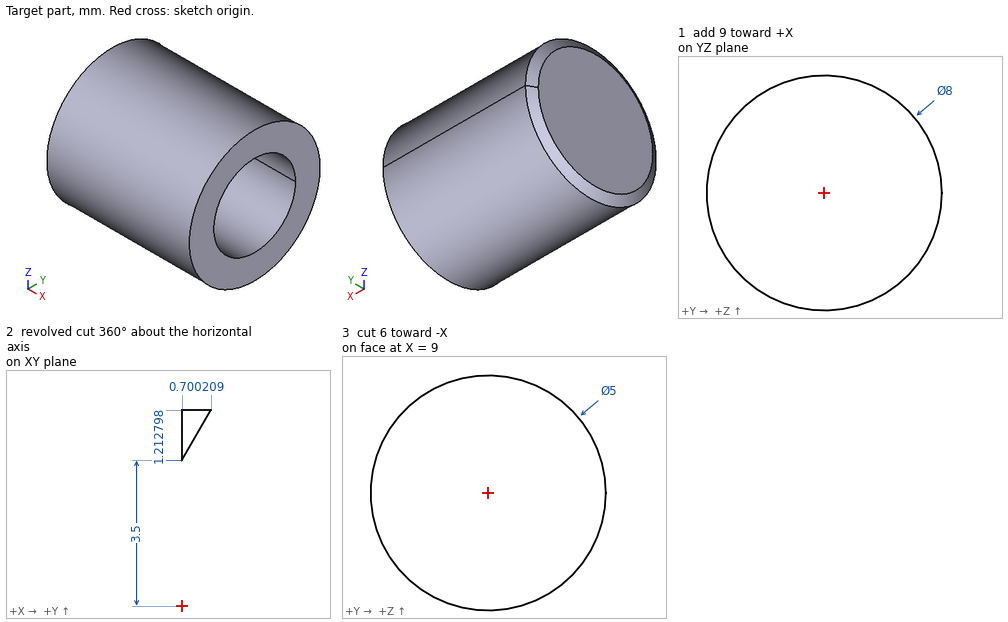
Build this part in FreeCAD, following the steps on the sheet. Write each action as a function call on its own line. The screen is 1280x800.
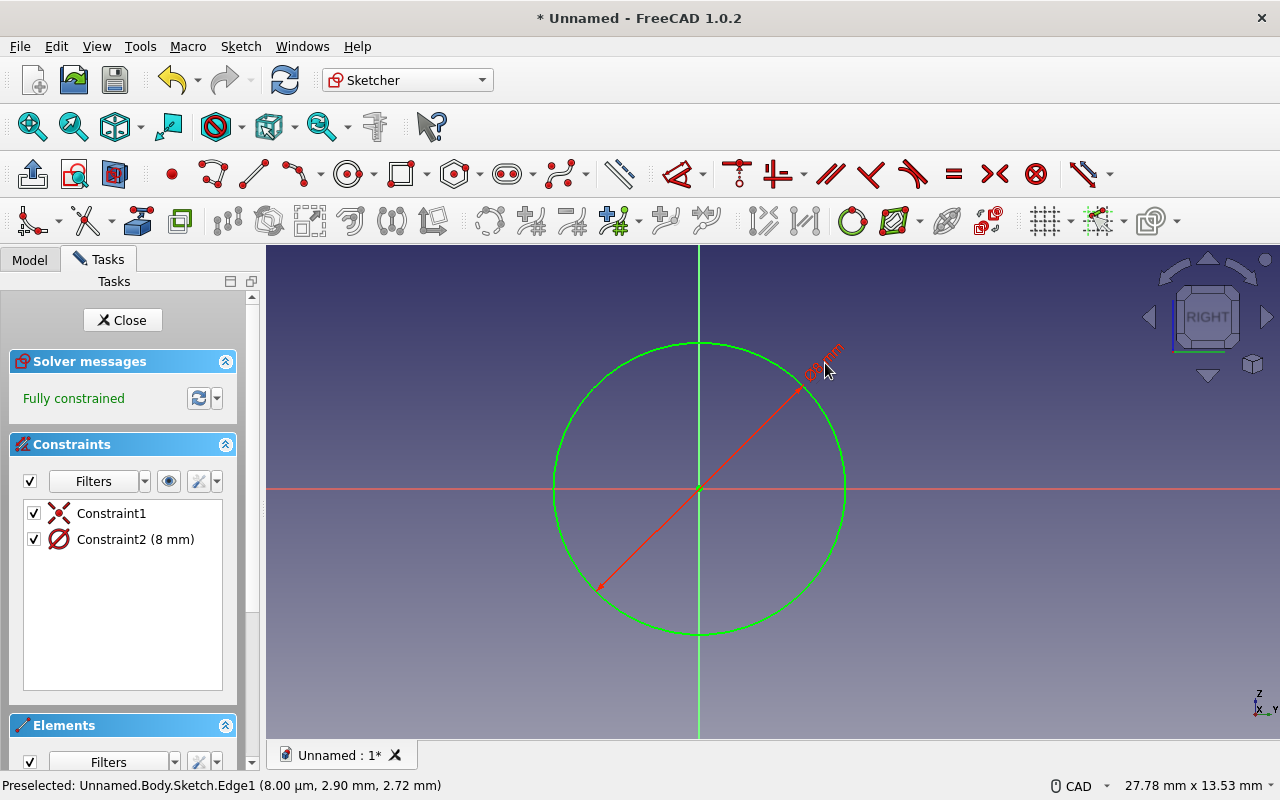
click(123, 320)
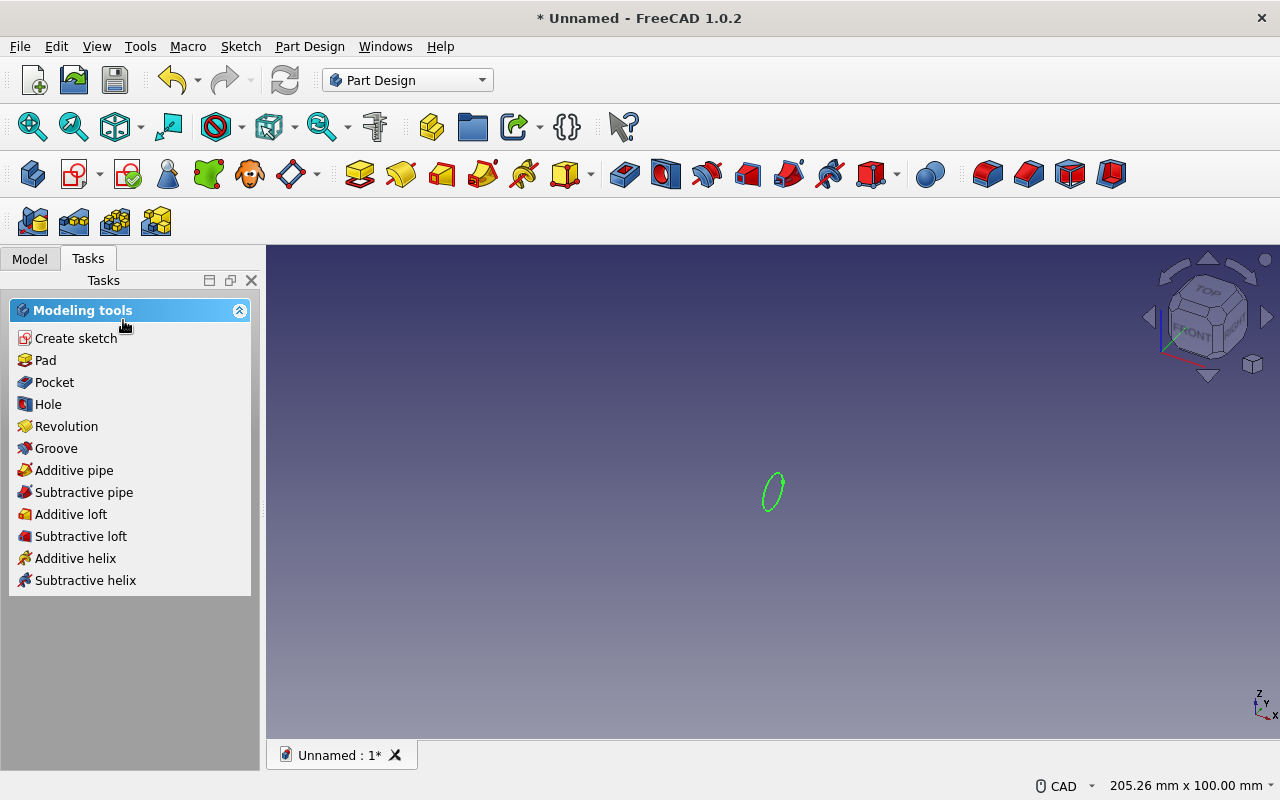
click(360, 174)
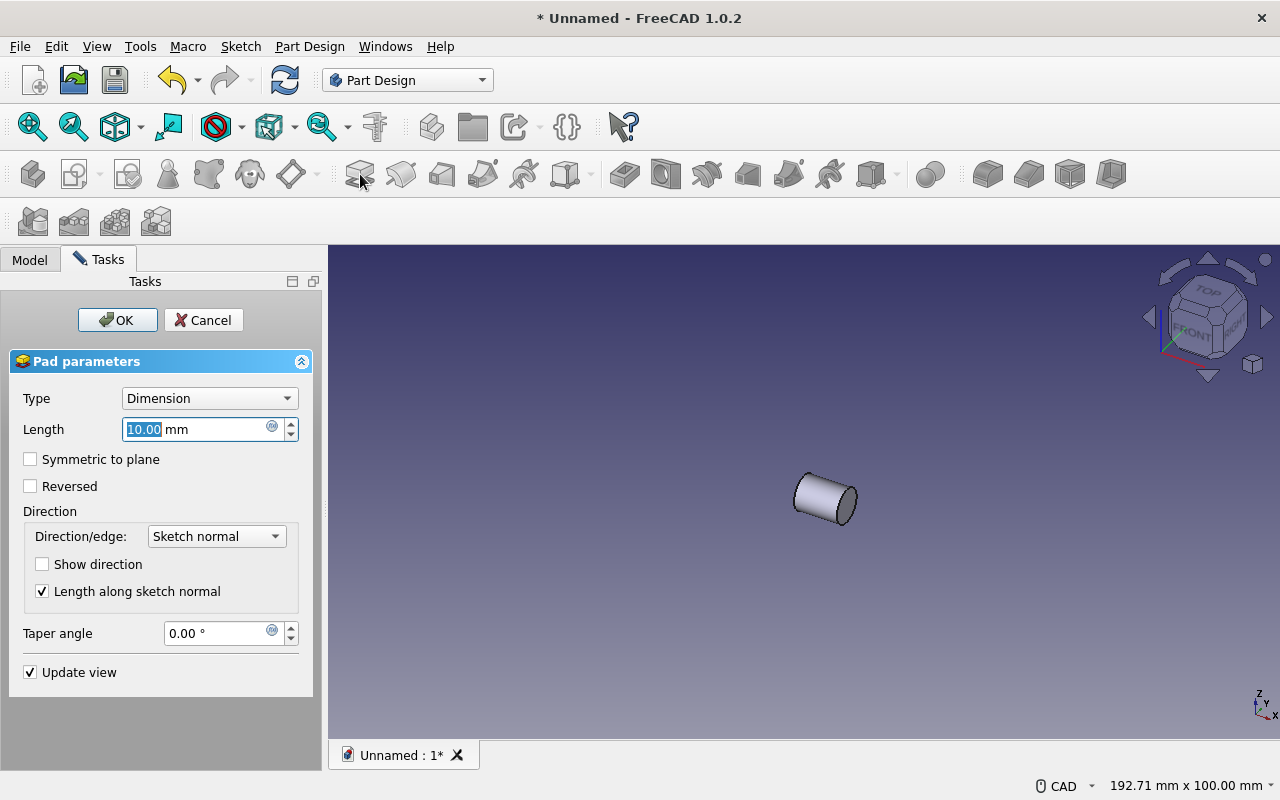
text(9)
key(Tab)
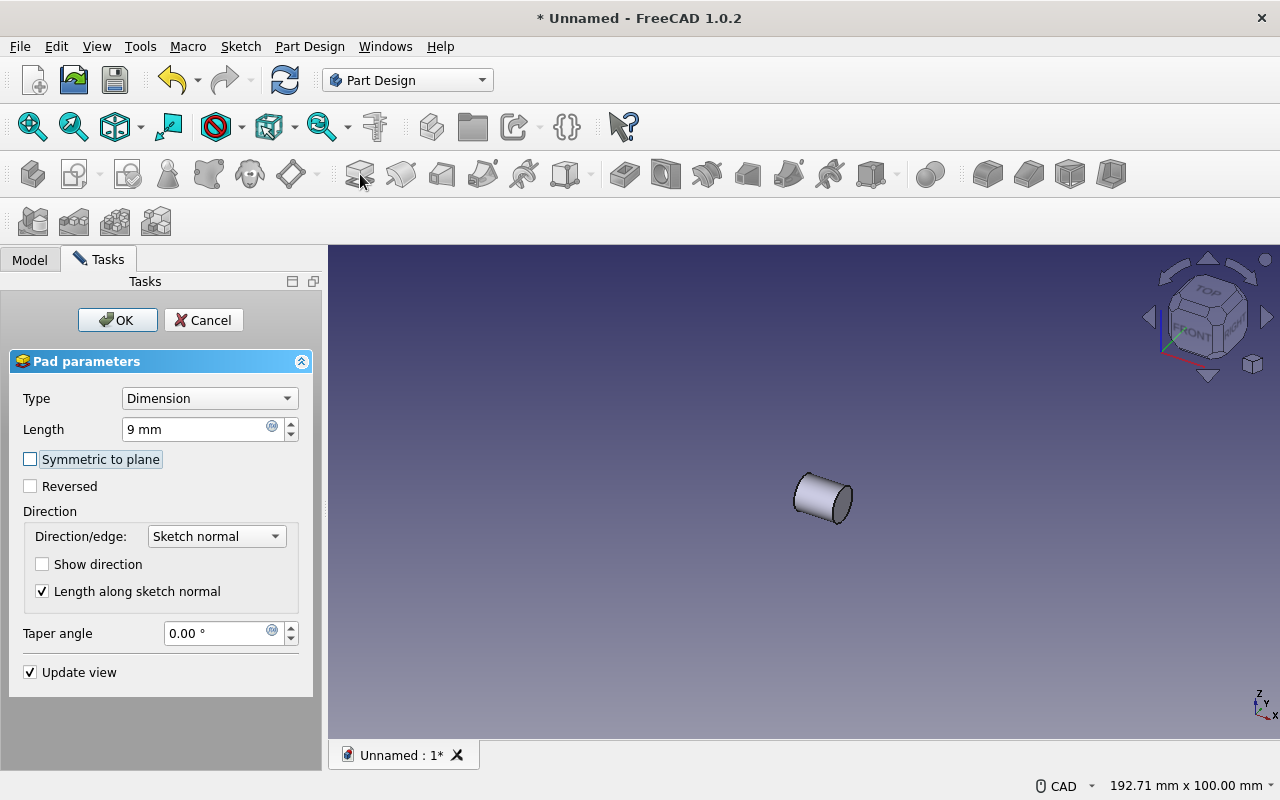
click(118, 320)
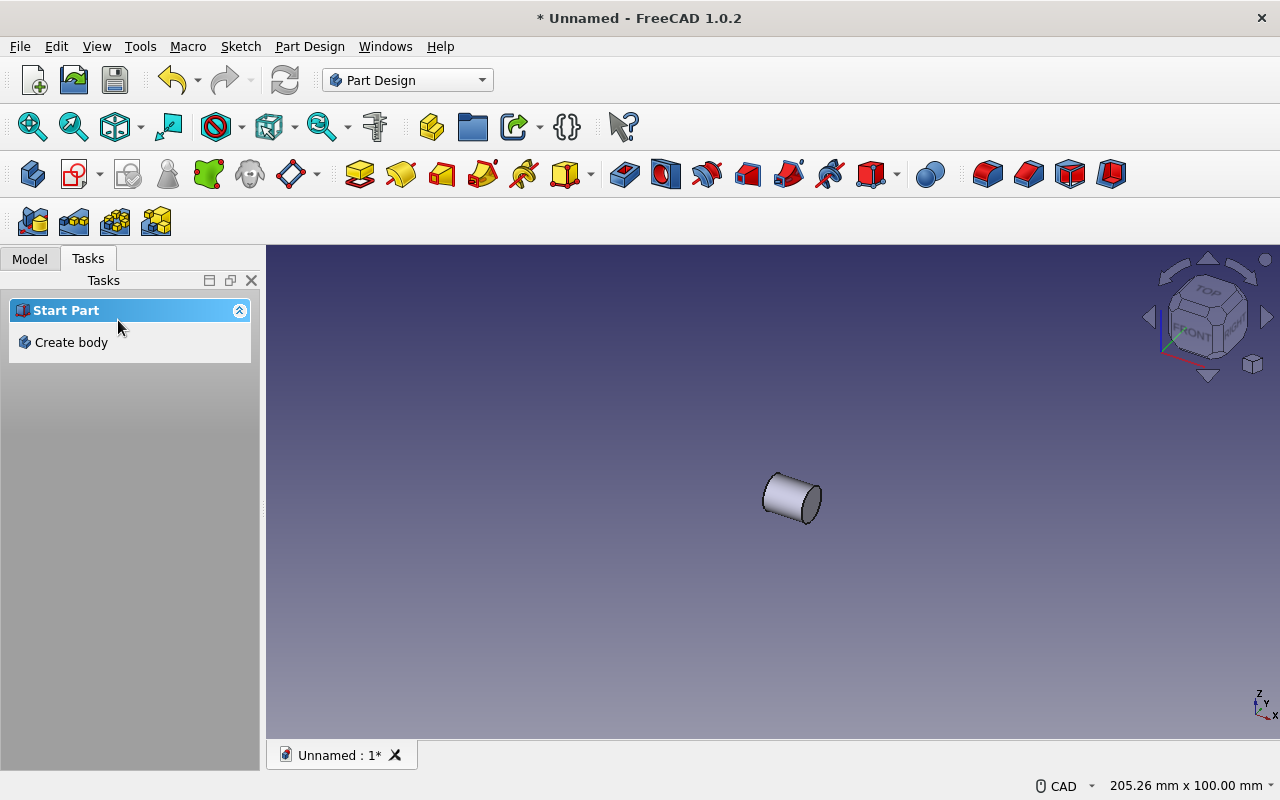
click(33, 128)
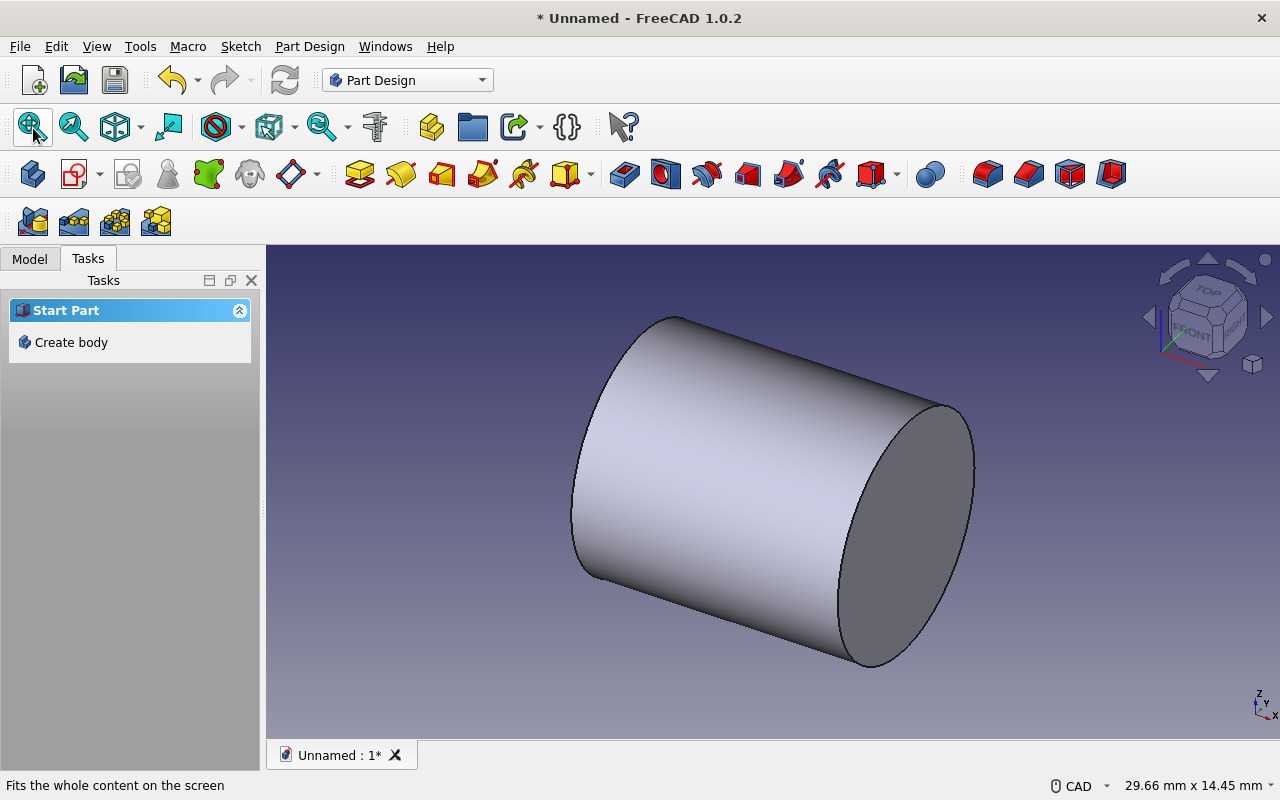
click(74, 174)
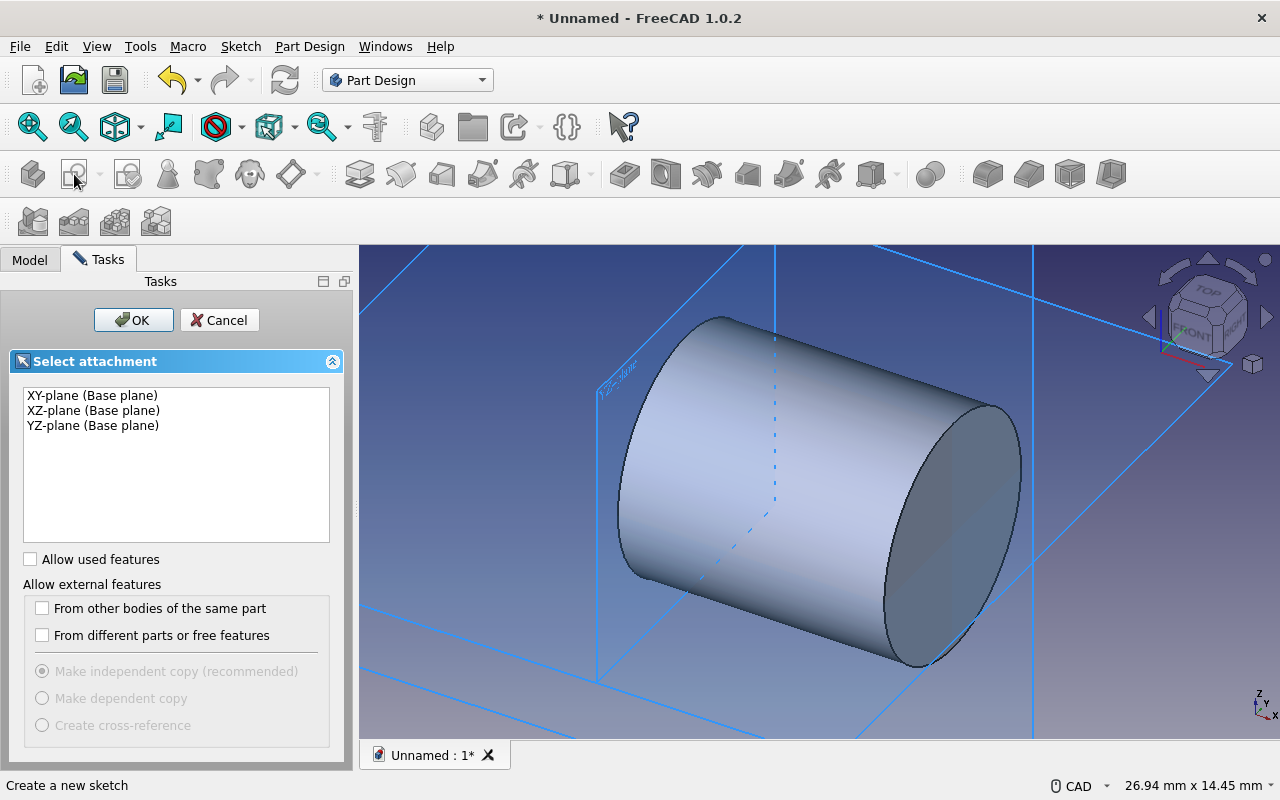
click(84, 396)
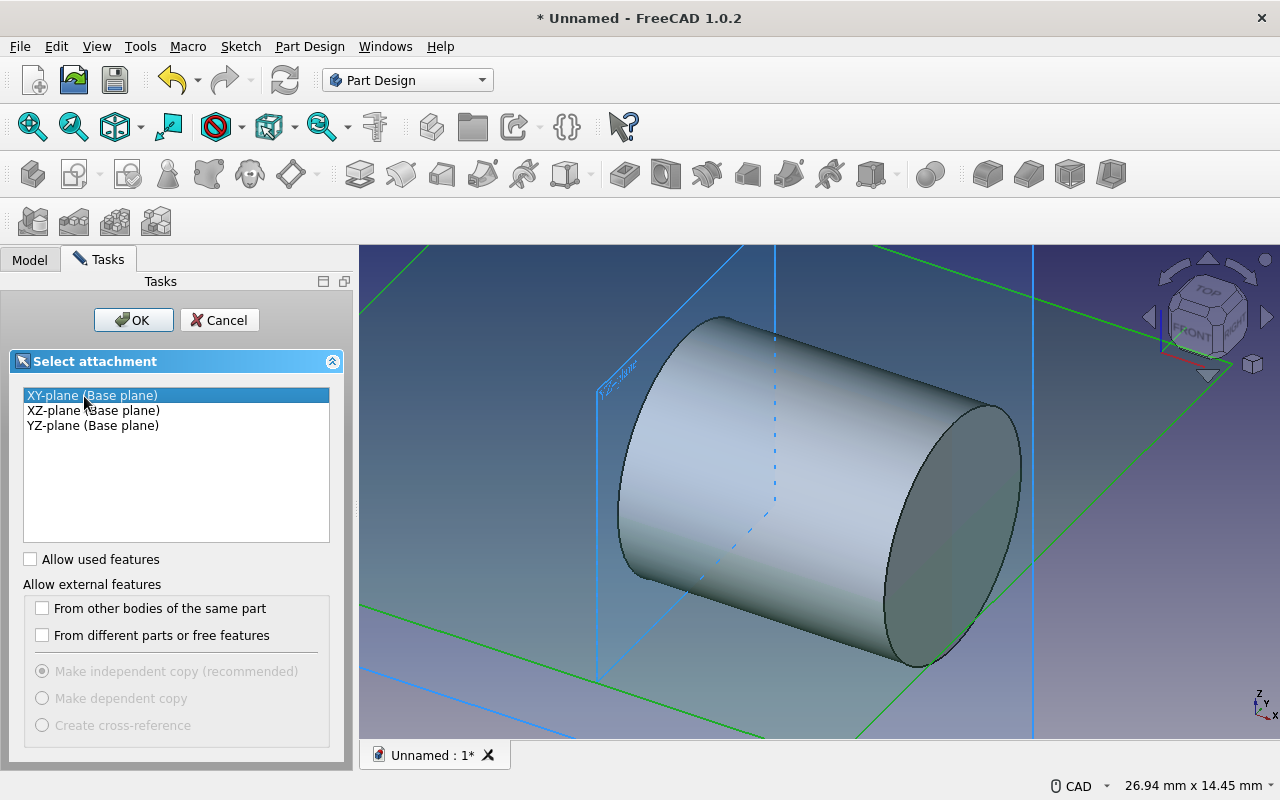
click(134, 320)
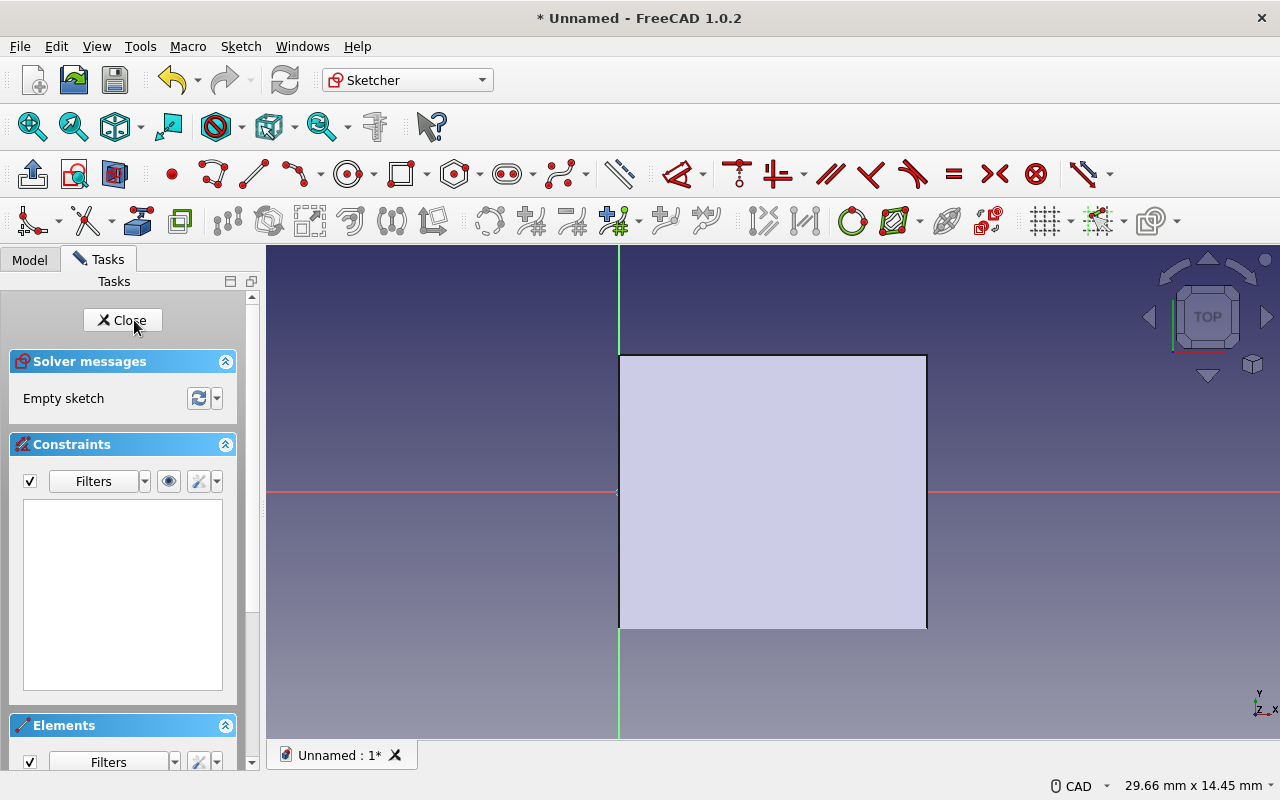
click(115, 174)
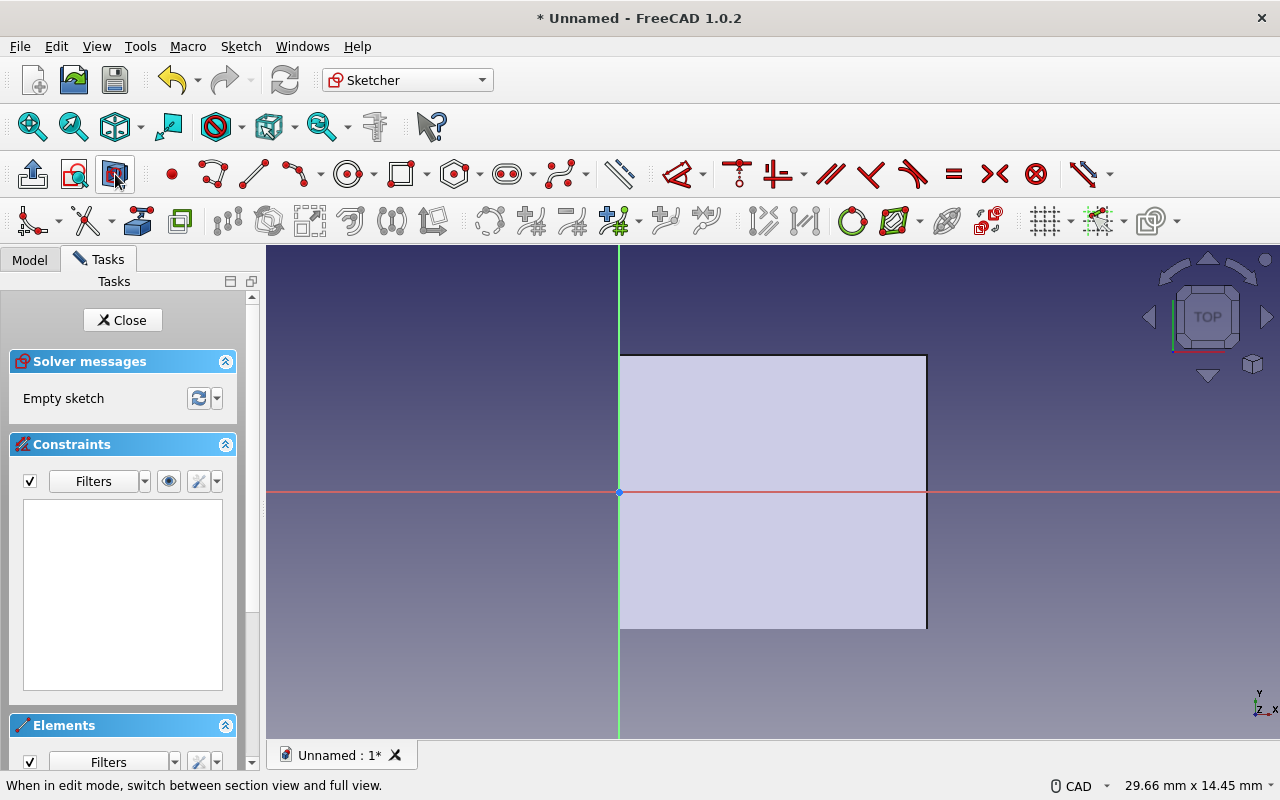
scroll(620, 330, up, 10)